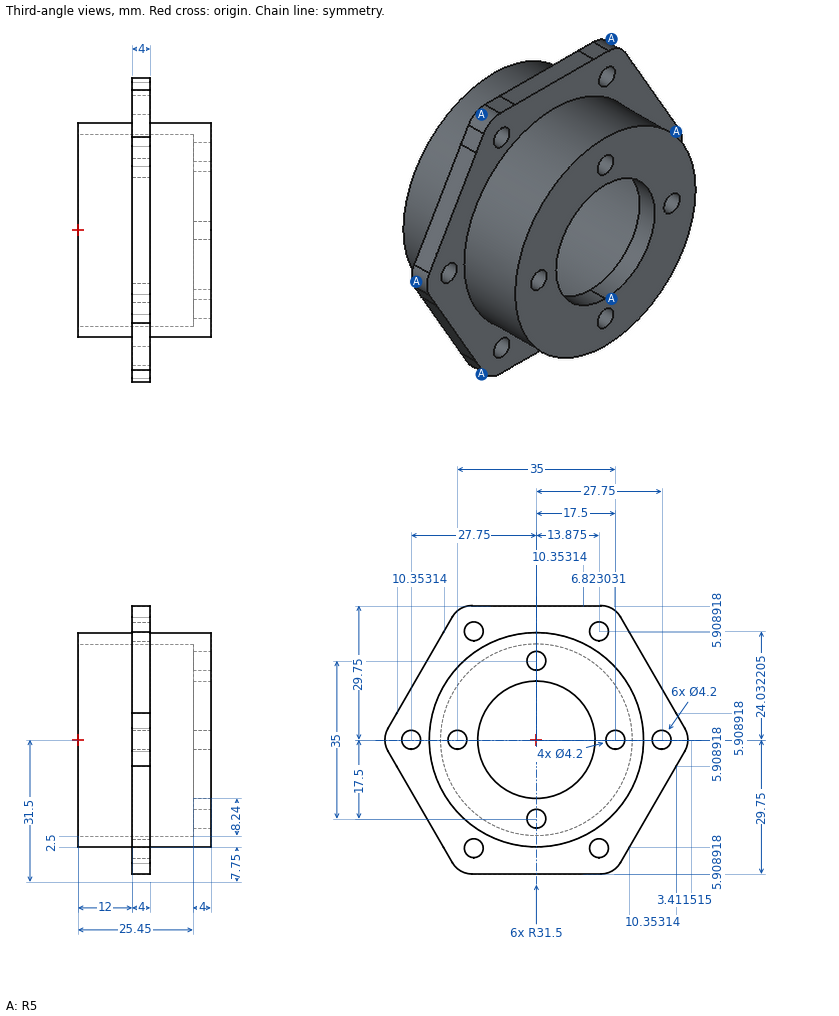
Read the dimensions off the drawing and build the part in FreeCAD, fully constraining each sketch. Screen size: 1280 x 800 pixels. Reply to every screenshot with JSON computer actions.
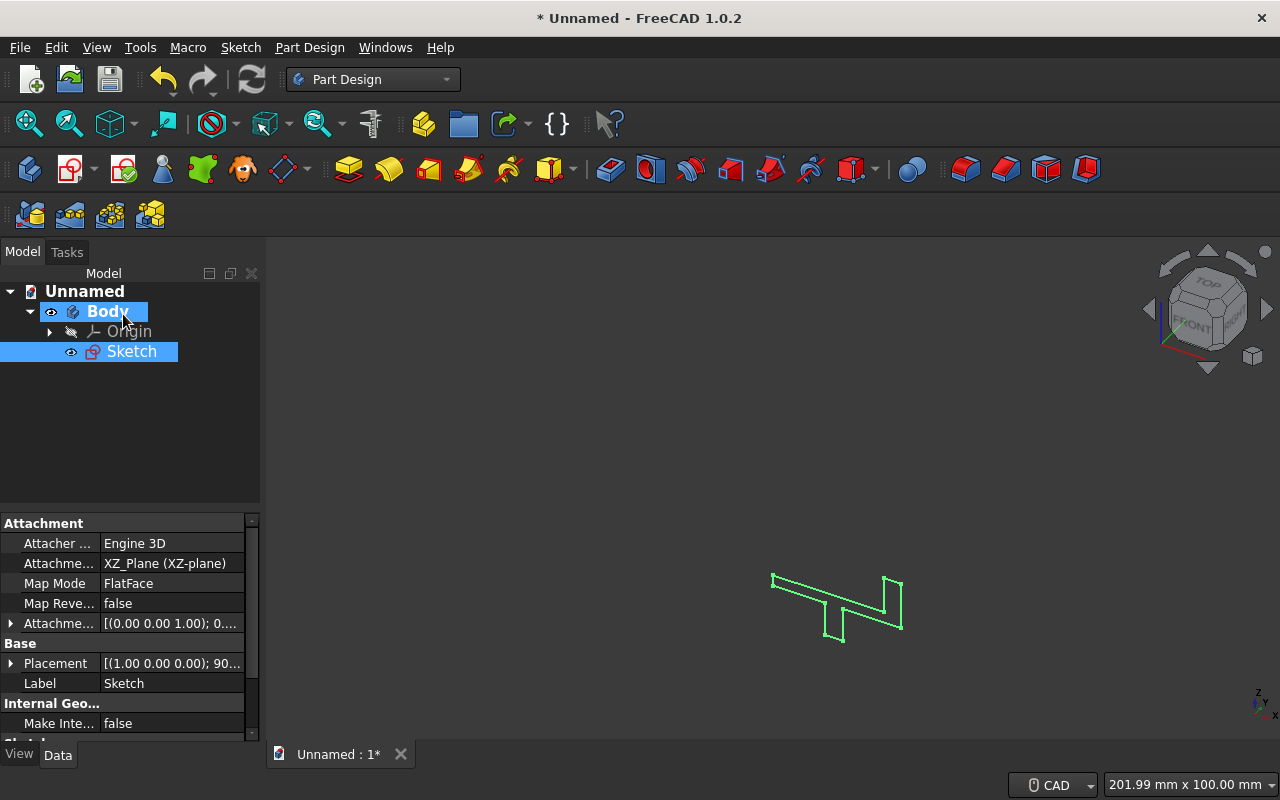
{"action": "left_click", "coordinate": [390, 170]}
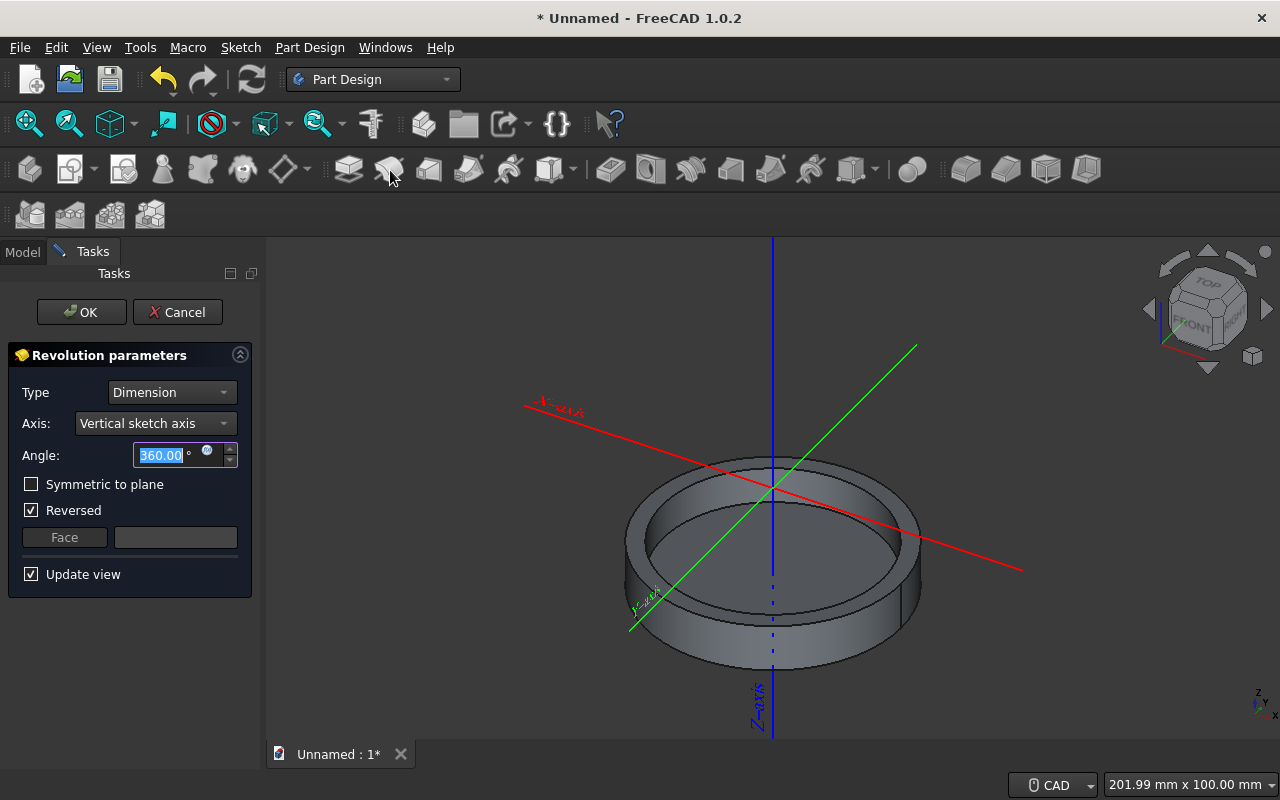
{"action": "left_click", "coordinate": [156, 424]}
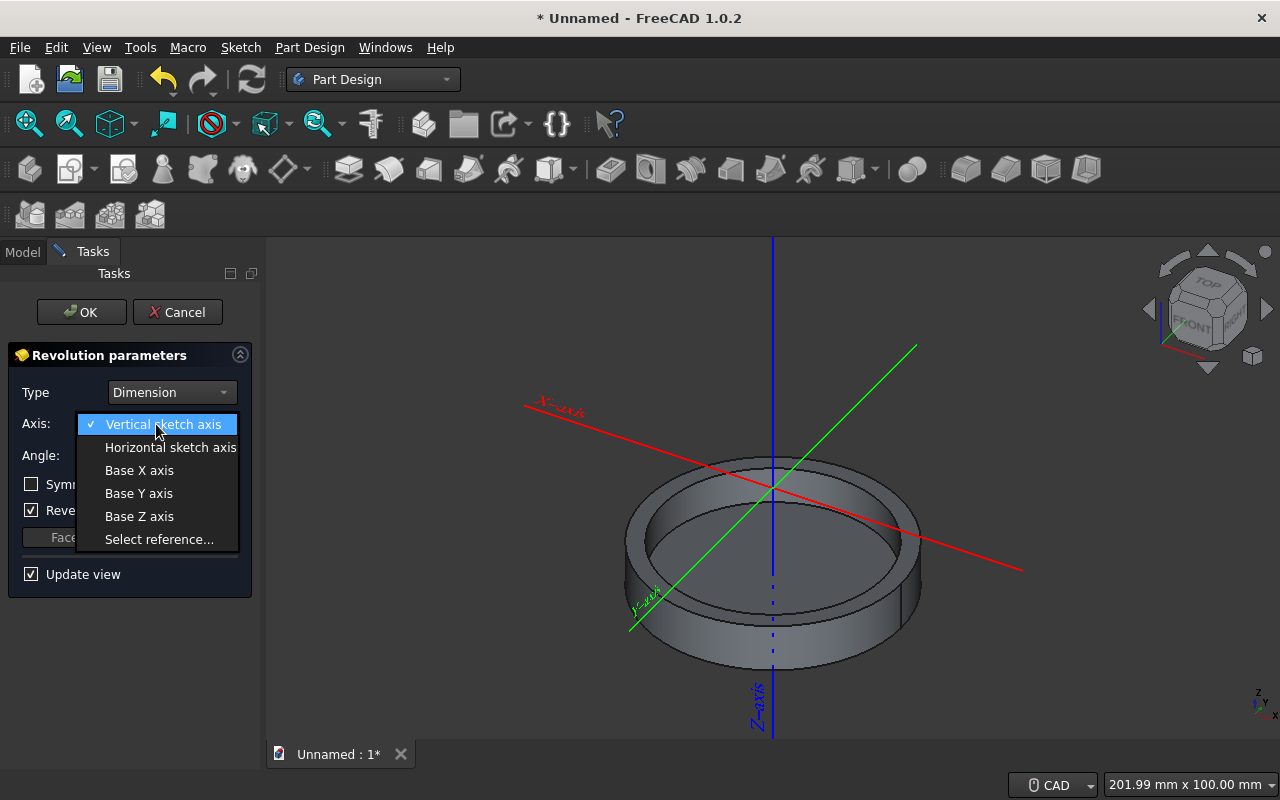
{"action": "left_click", "coordinate": [156, 448]}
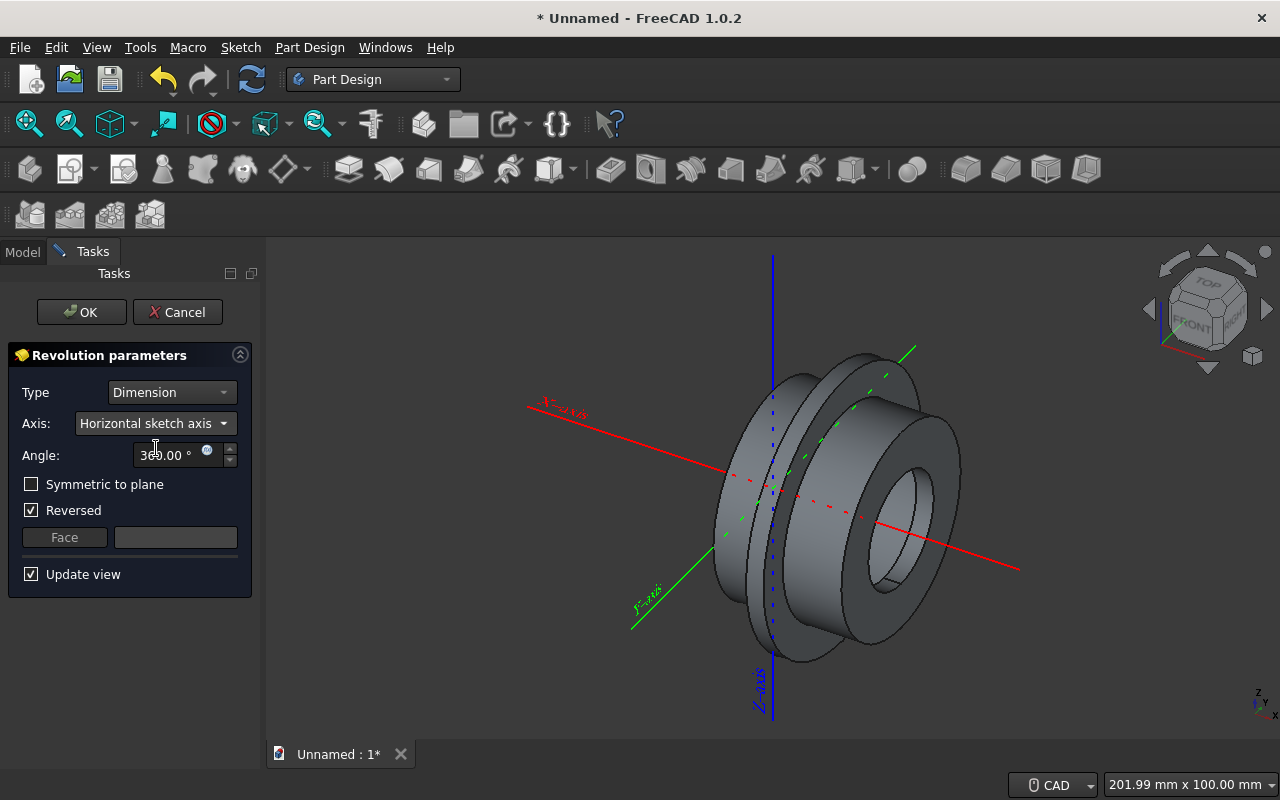
{"action": "left_click", "coordinate": [82, 312]}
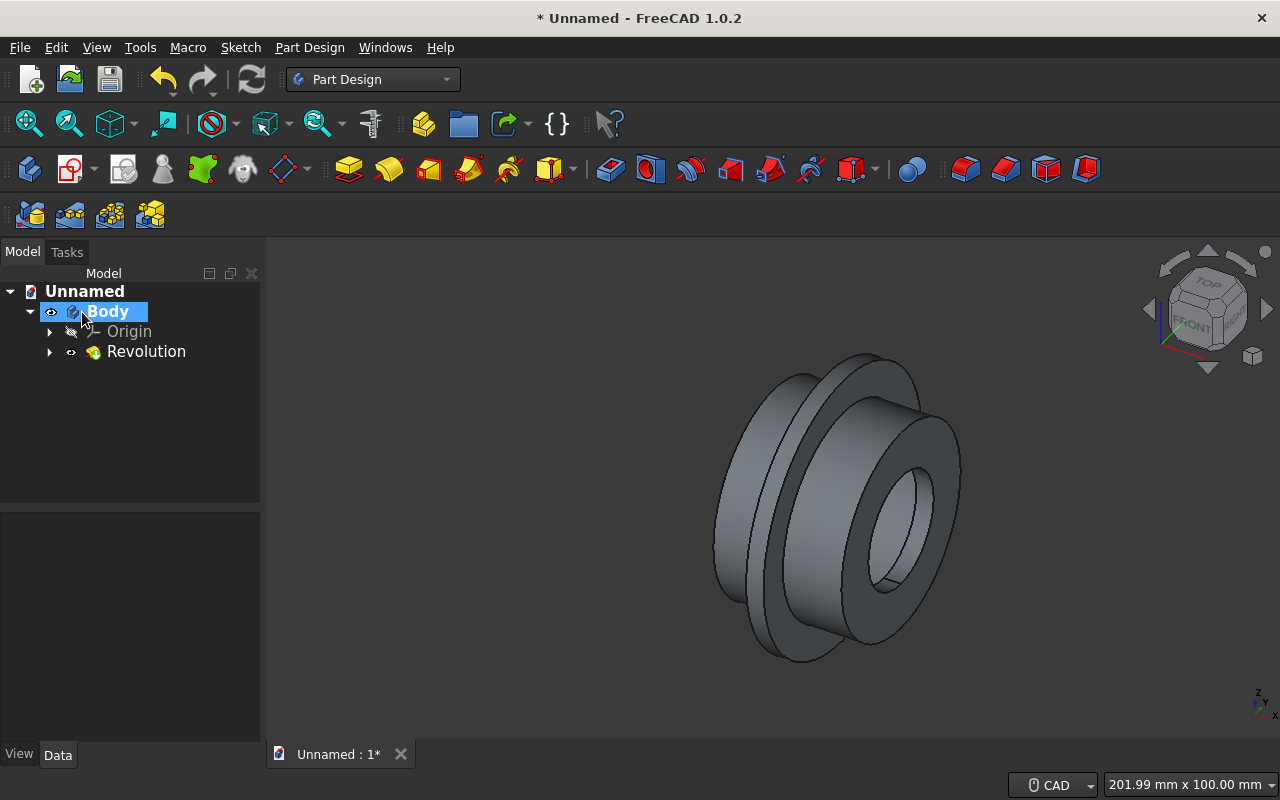
{"action": "left_click", "coordinate": [843, 399]}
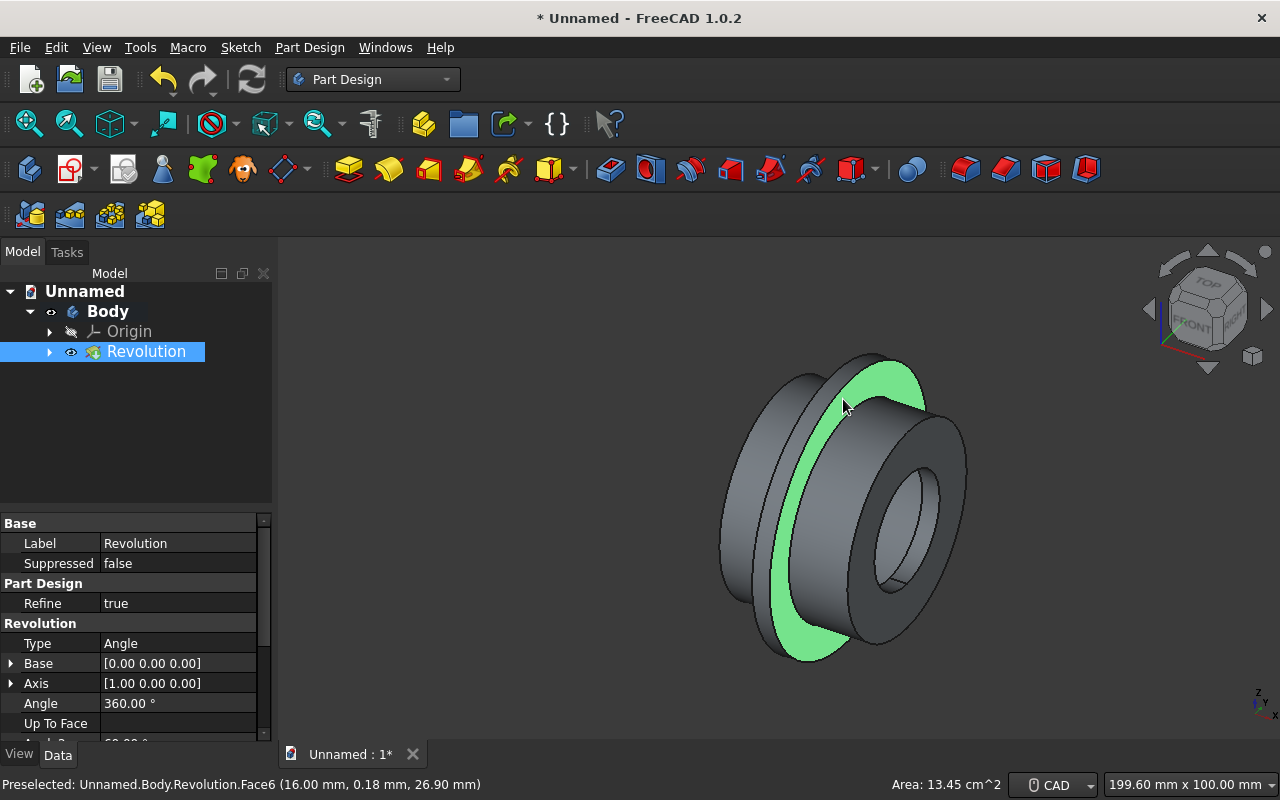
{"action": "left_click", "coordinate": [70, 170]}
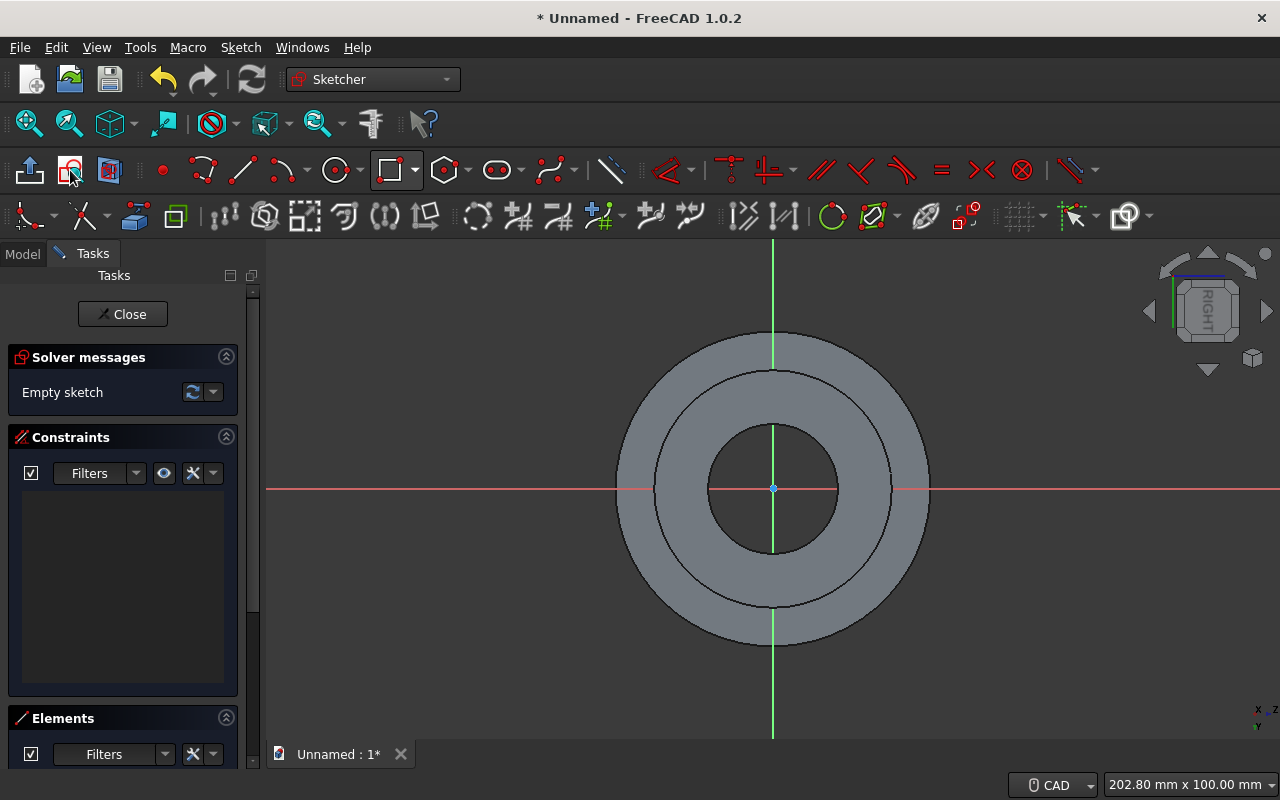
{"action": "key", "text": "g l"}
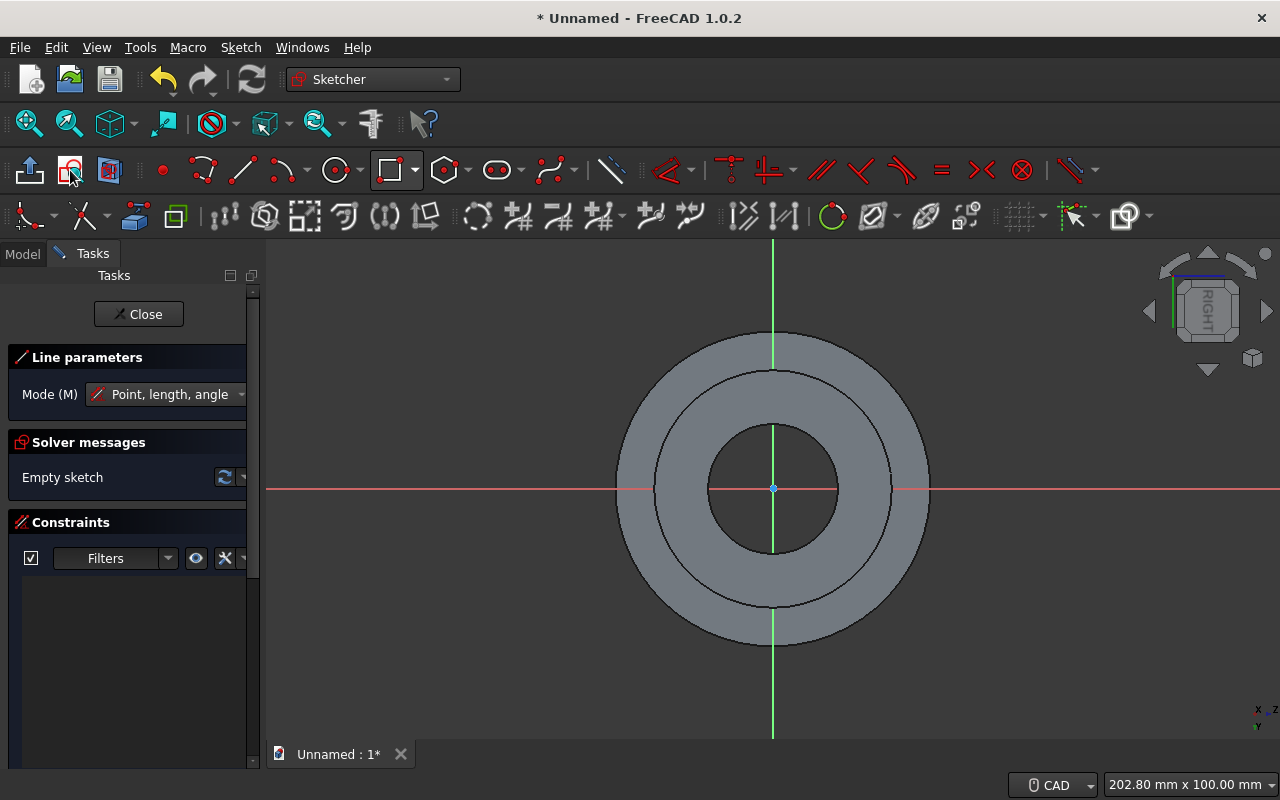
{"action": "left_click", "coordinate": [624, 541]}
{"action": "left_click", "coordinate": [624, 437]}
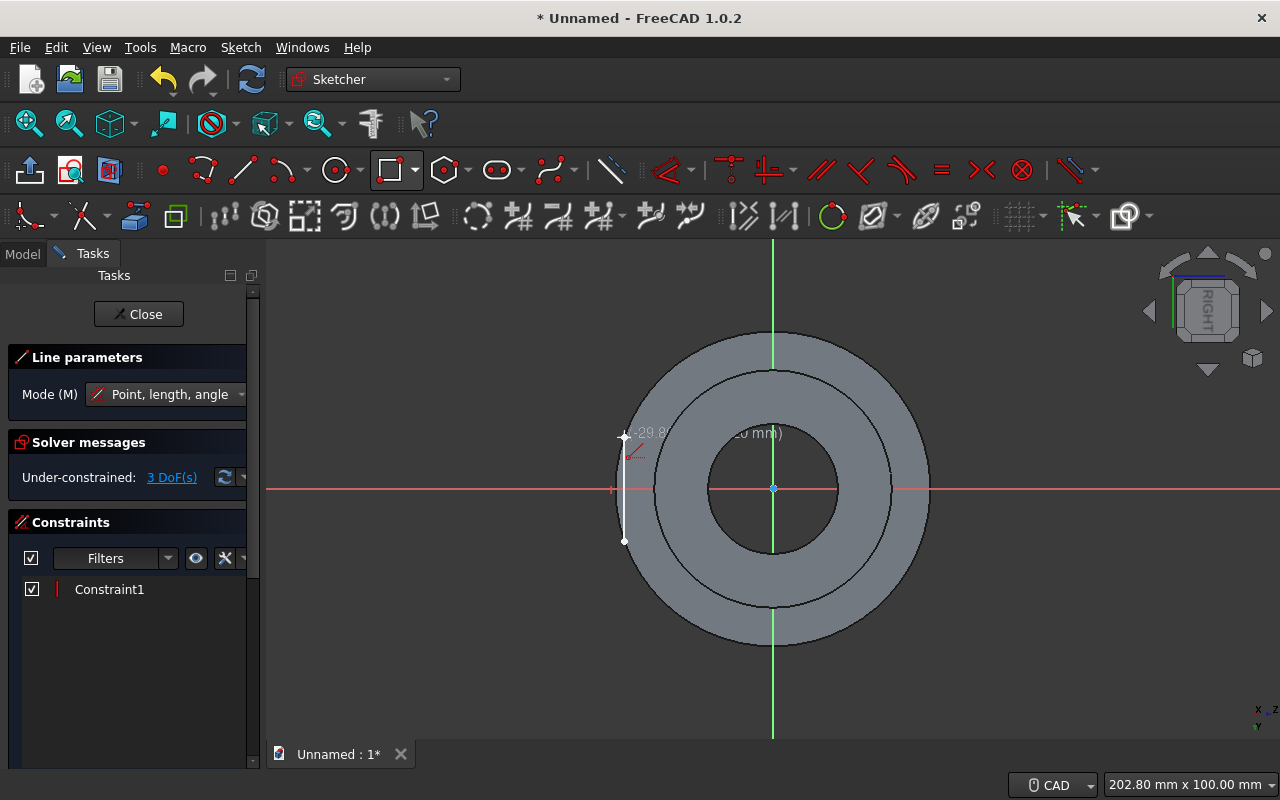
{"action": "key", "text": "g 3 a"}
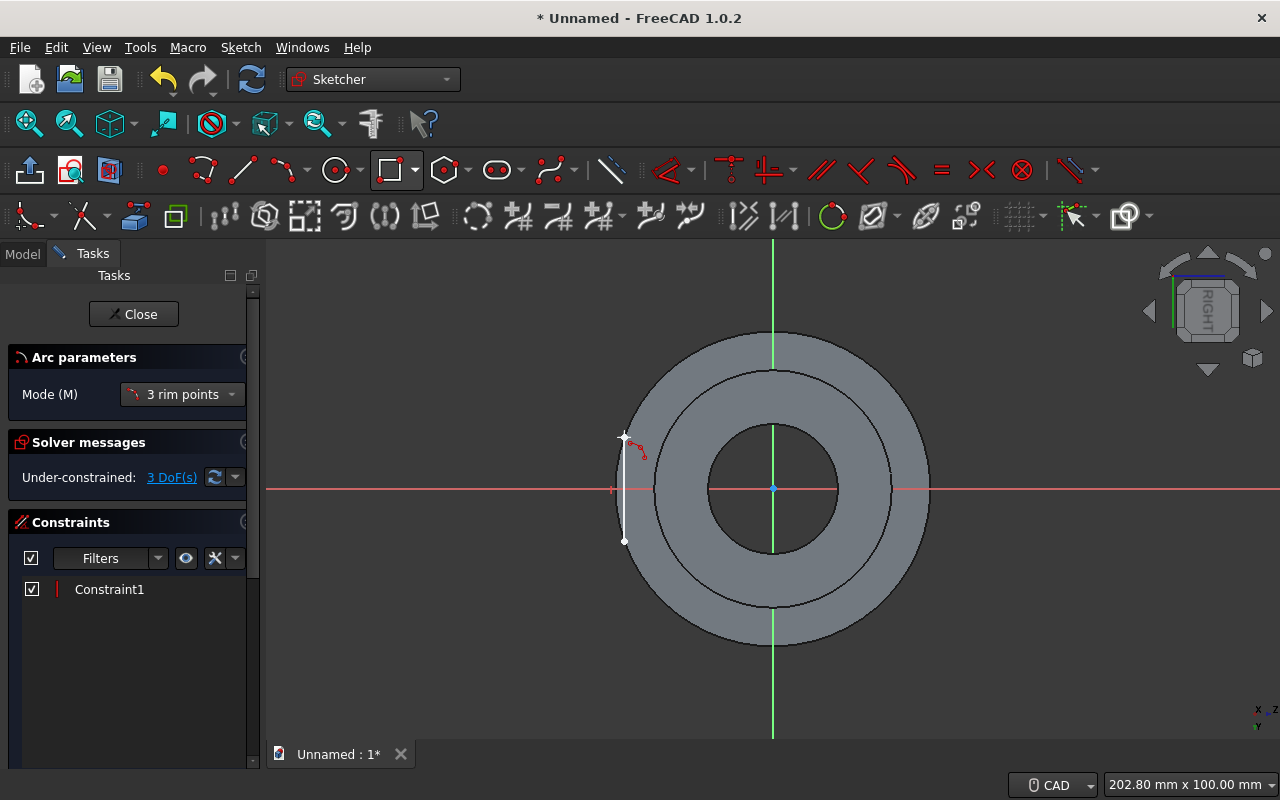
{"action": "left_click", "coordinate": [624, 438]}
{"action": "left_click", "coordinate": [624, 542]}